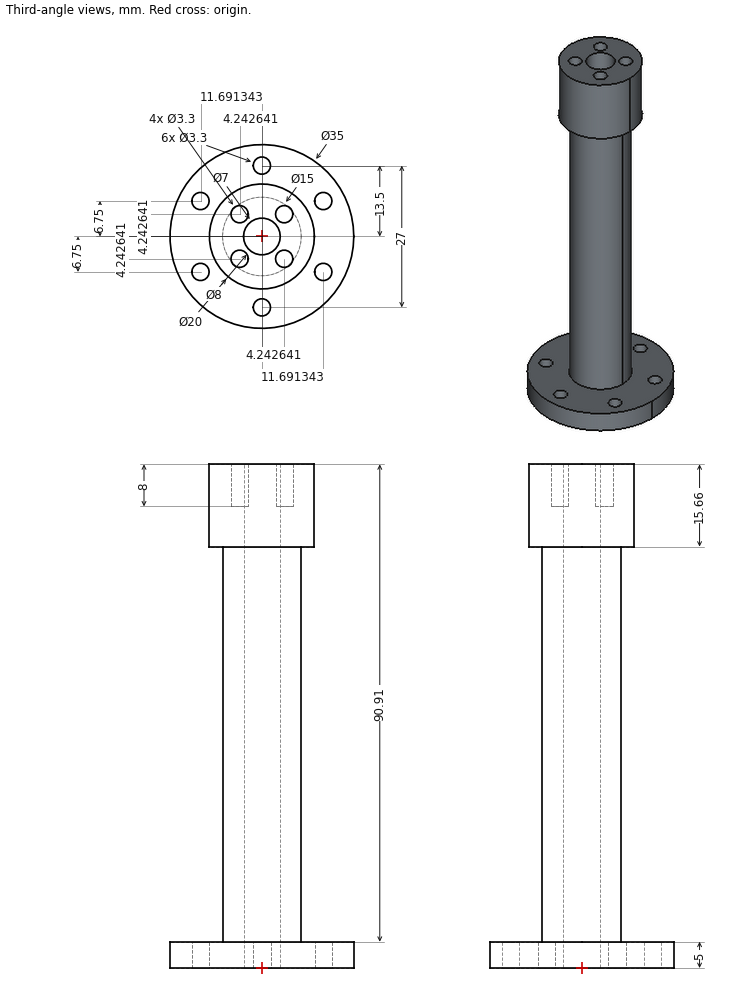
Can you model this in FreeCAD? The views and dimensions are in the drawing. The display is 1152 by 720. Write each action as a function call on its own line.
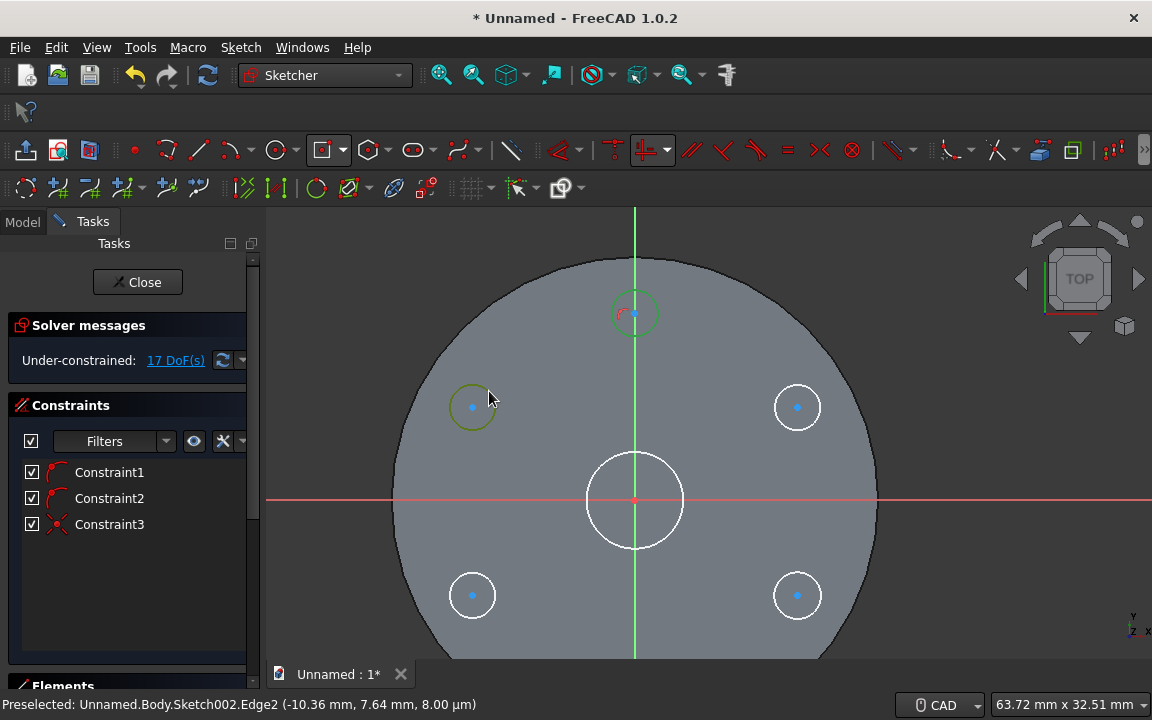
click(489, 579)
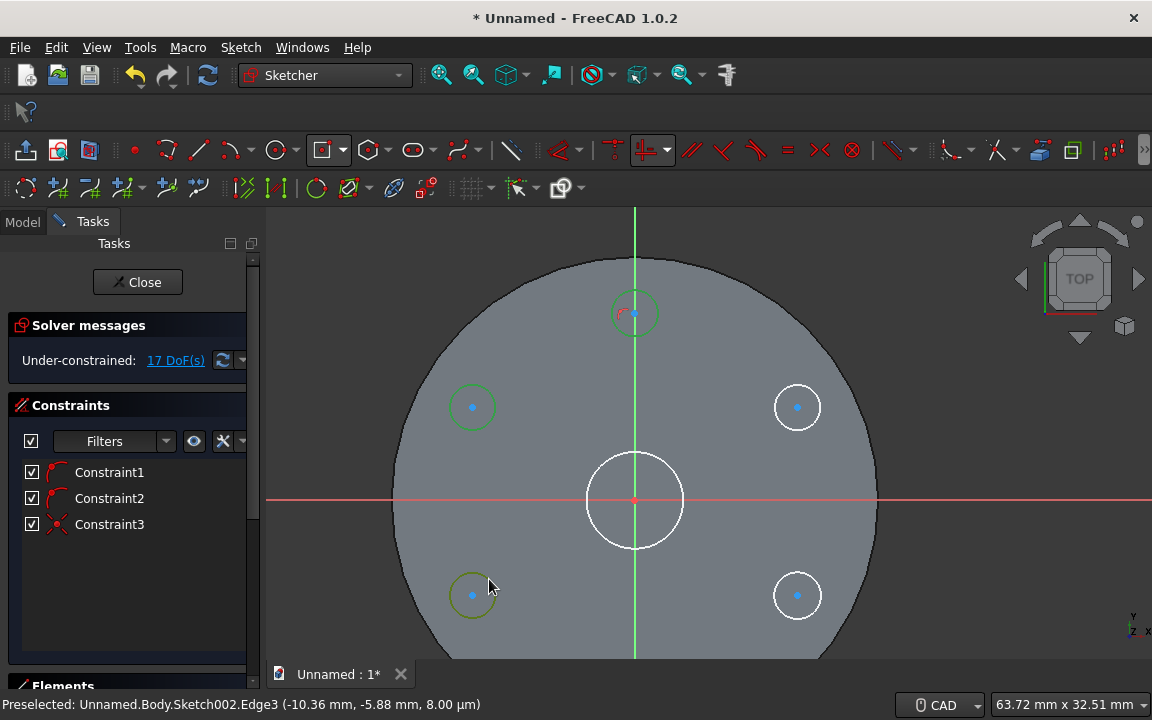
scroll(652, 296, down, 2)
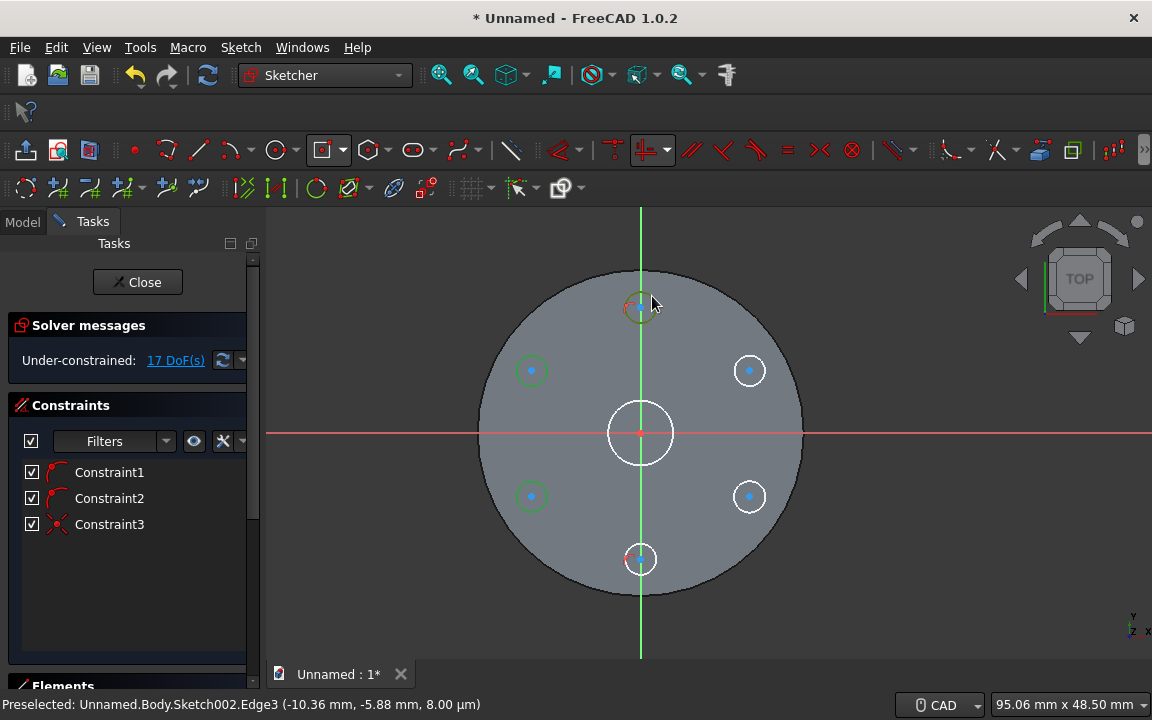
scroll(652, 548, up, 2)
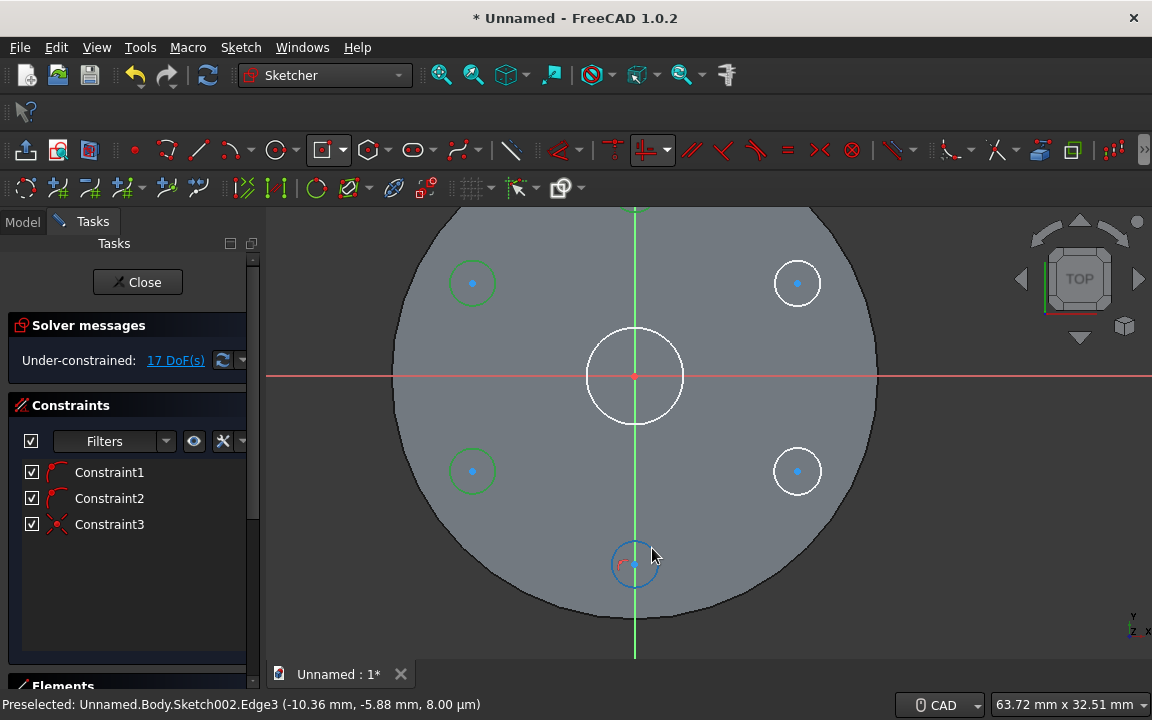
click(651, 548)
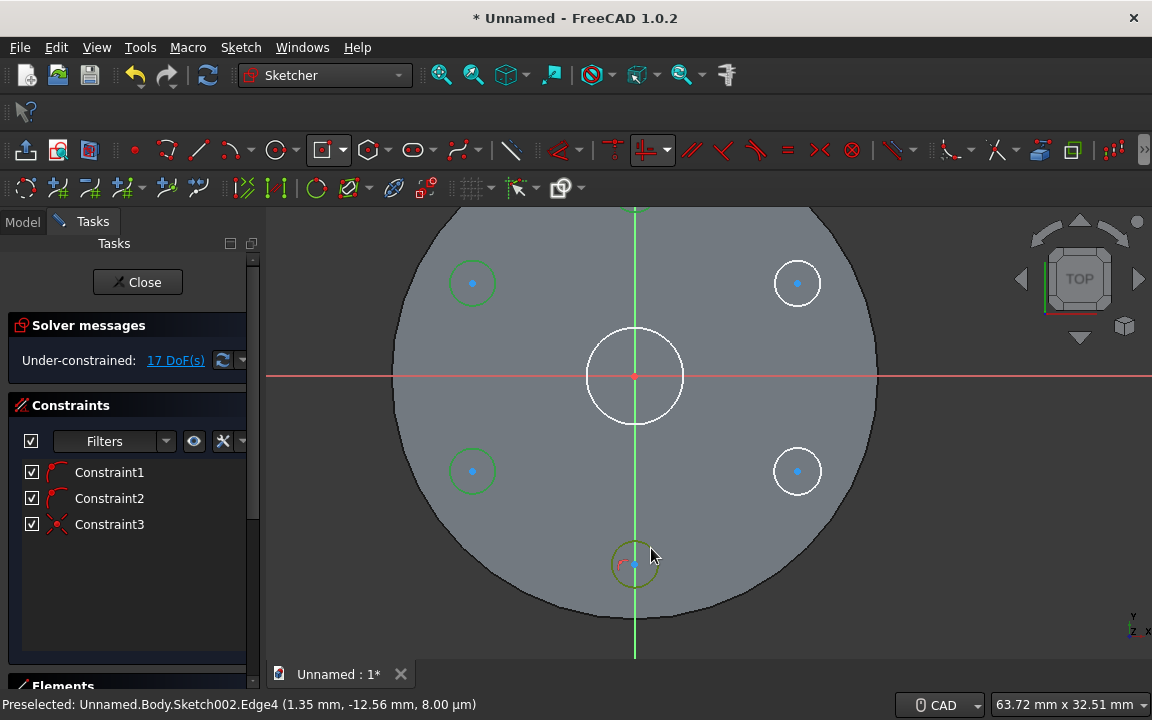
click(814, 455)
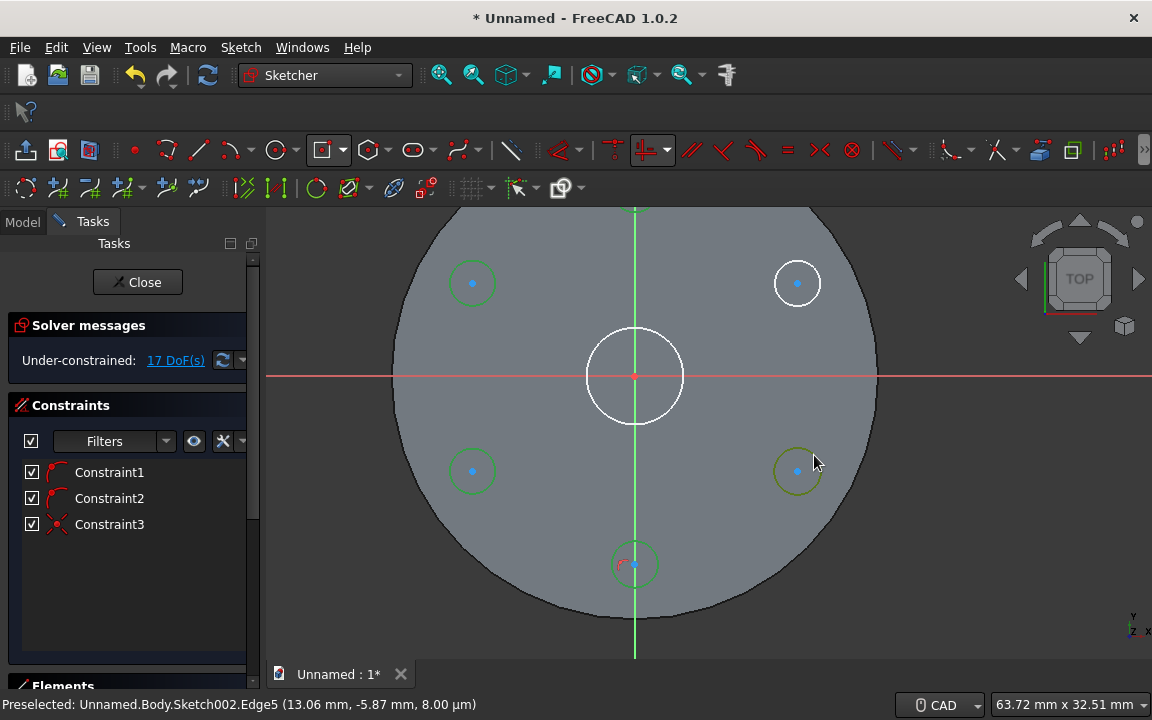
click(814, 267)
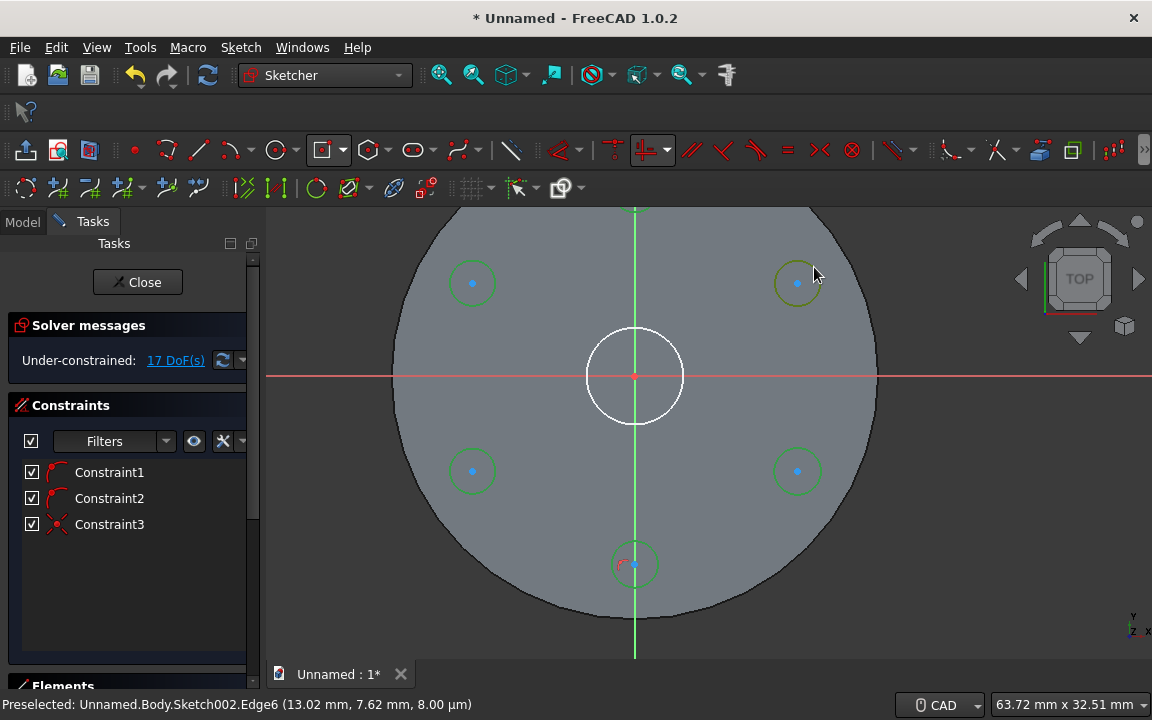
key(e)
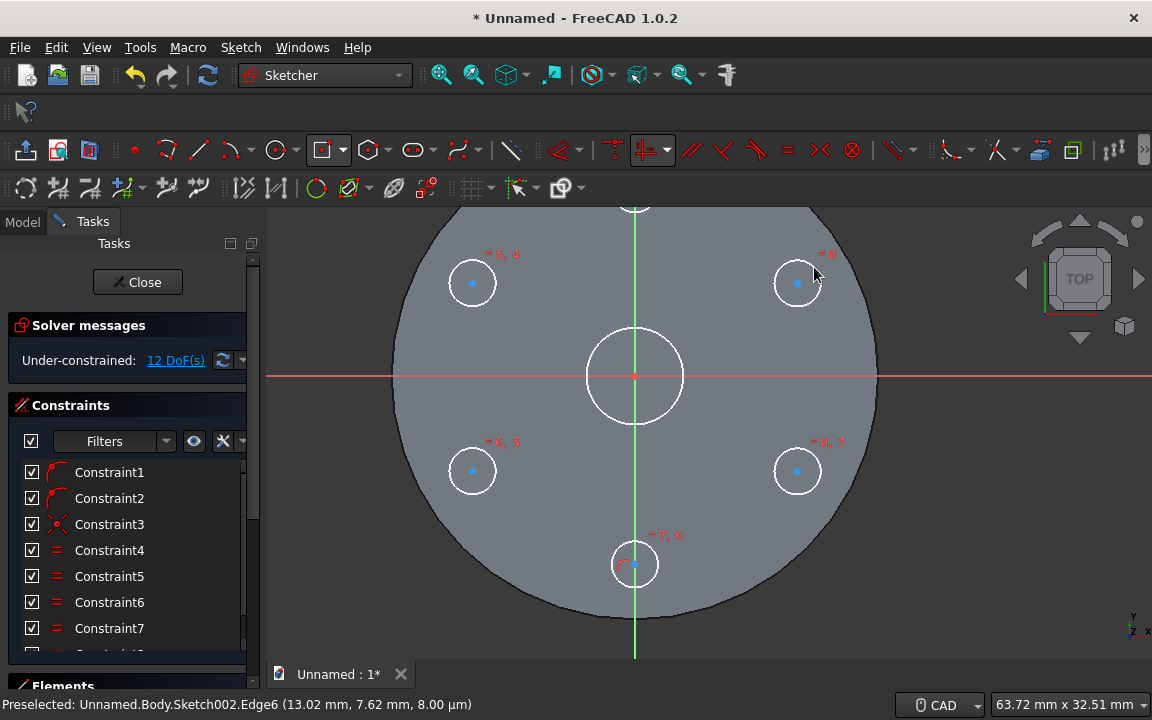
click(473, 283)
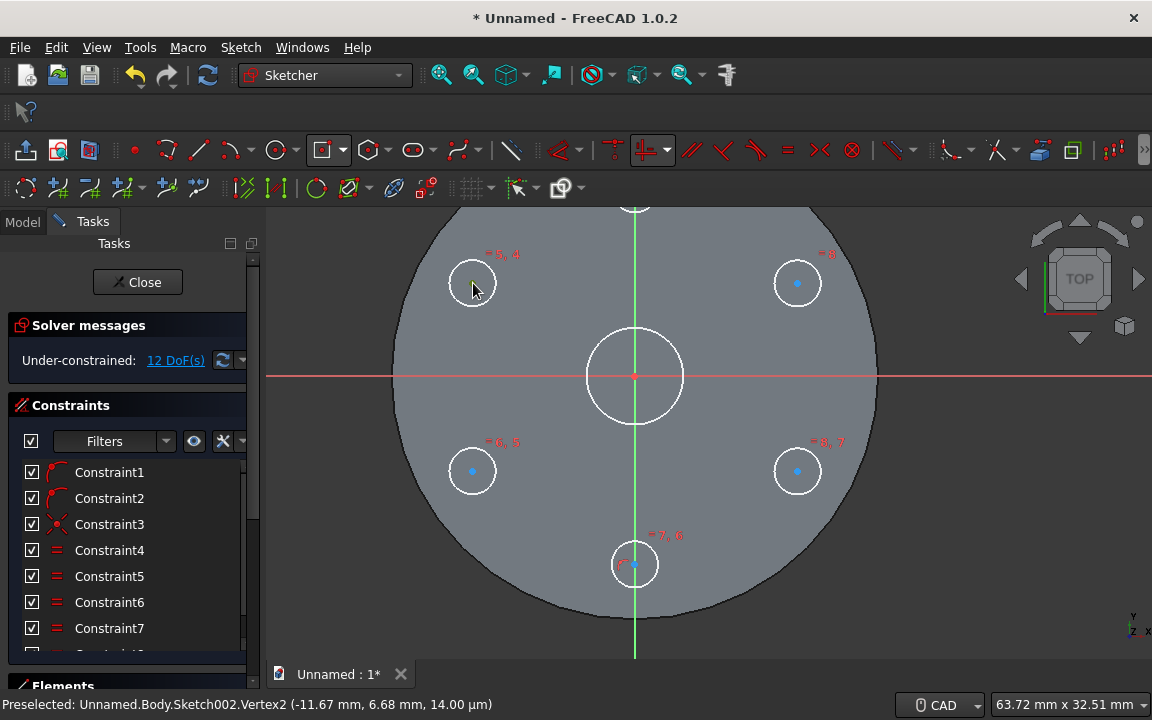
click(473, 471)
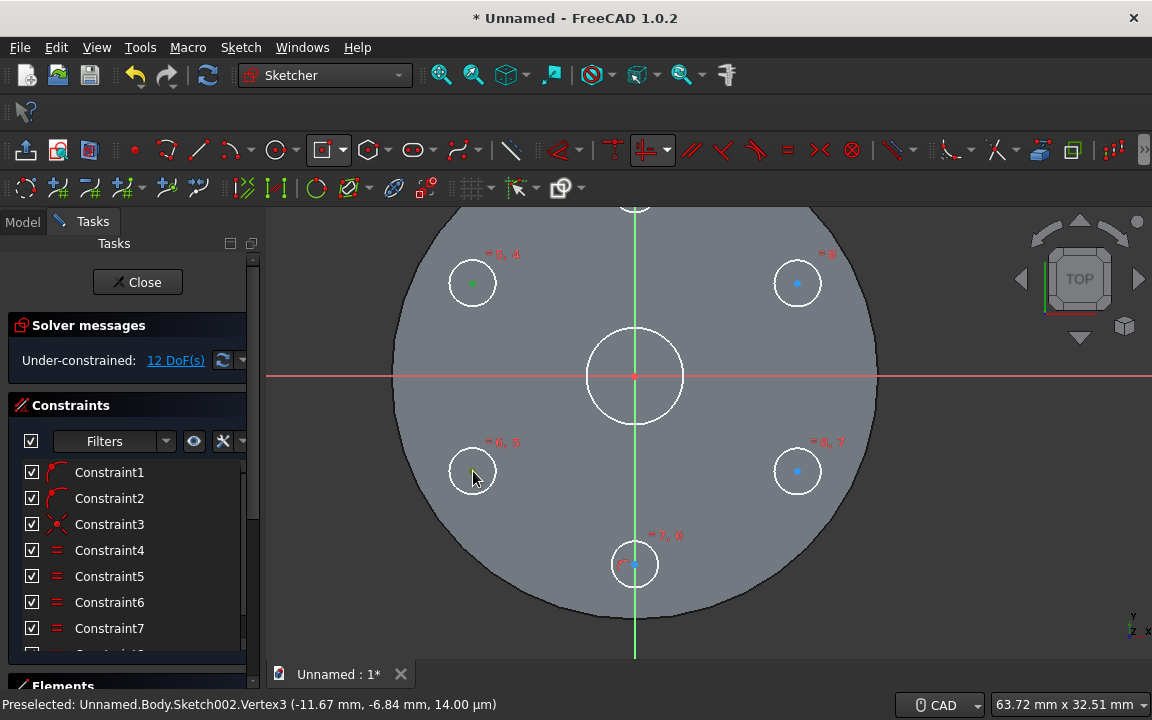
key(v)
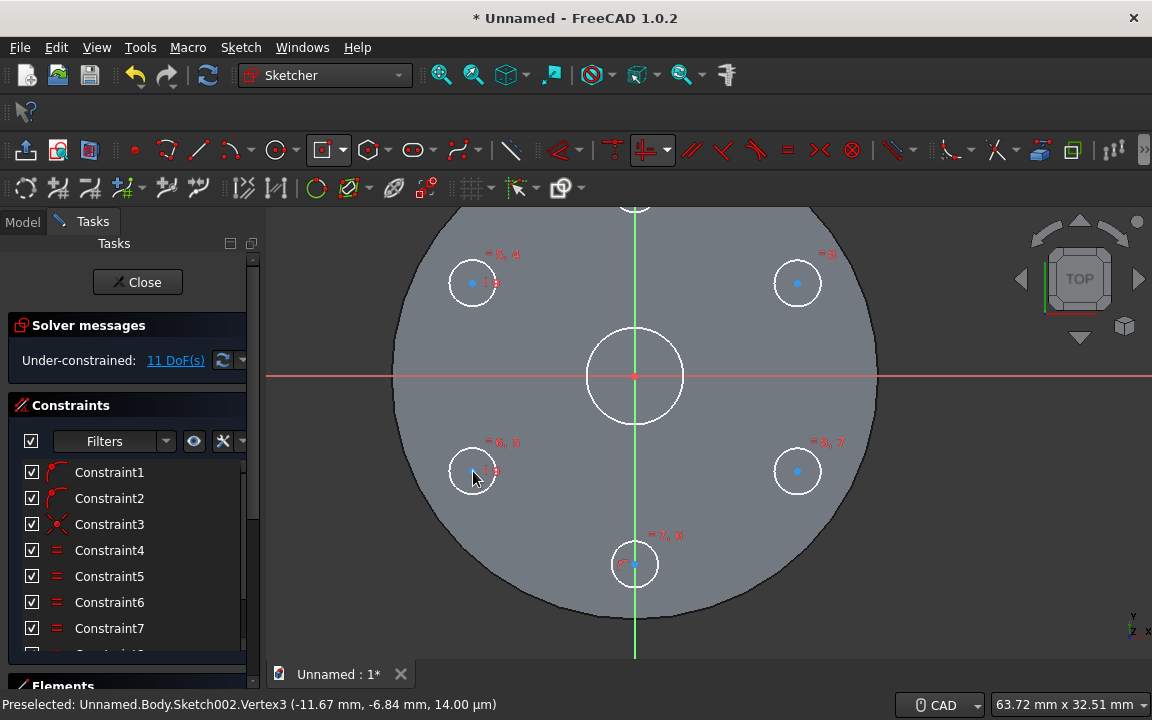
click(473, 471)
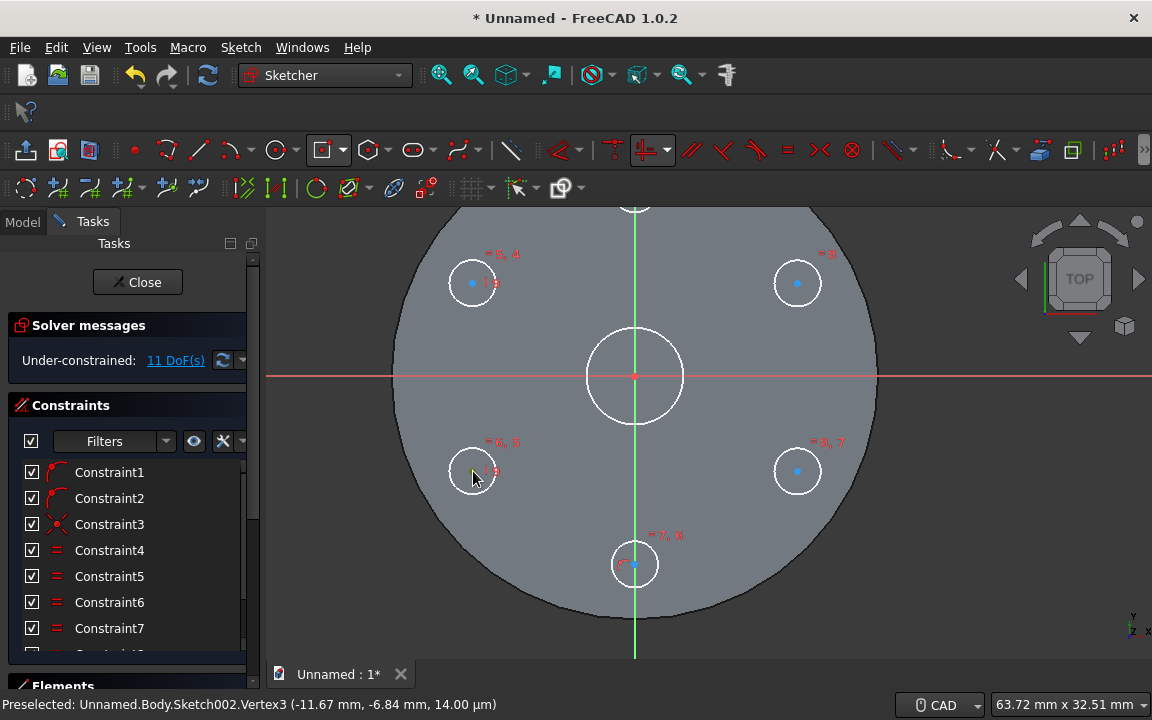
click(798, 471)